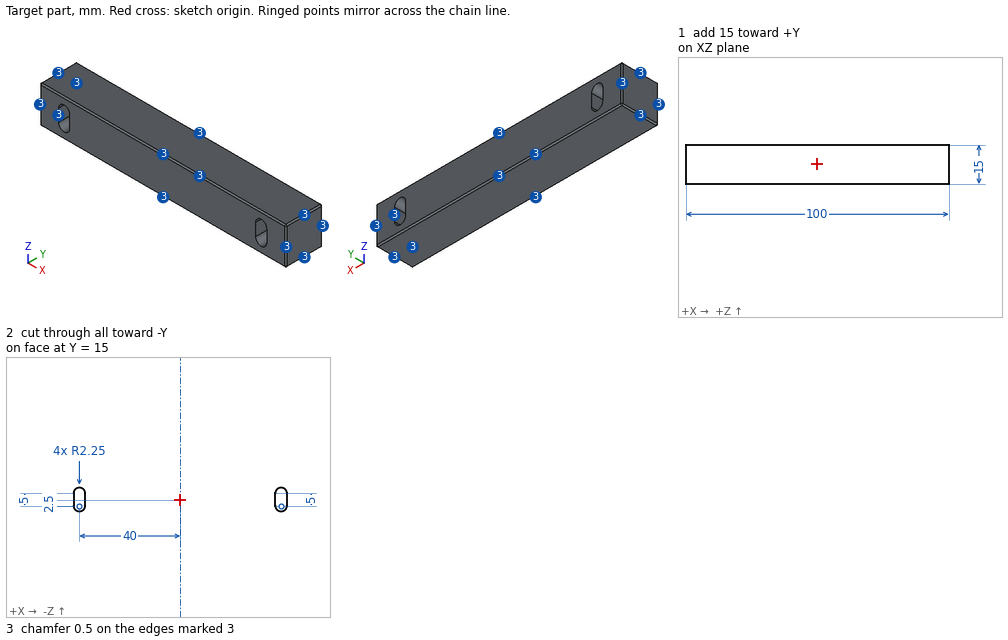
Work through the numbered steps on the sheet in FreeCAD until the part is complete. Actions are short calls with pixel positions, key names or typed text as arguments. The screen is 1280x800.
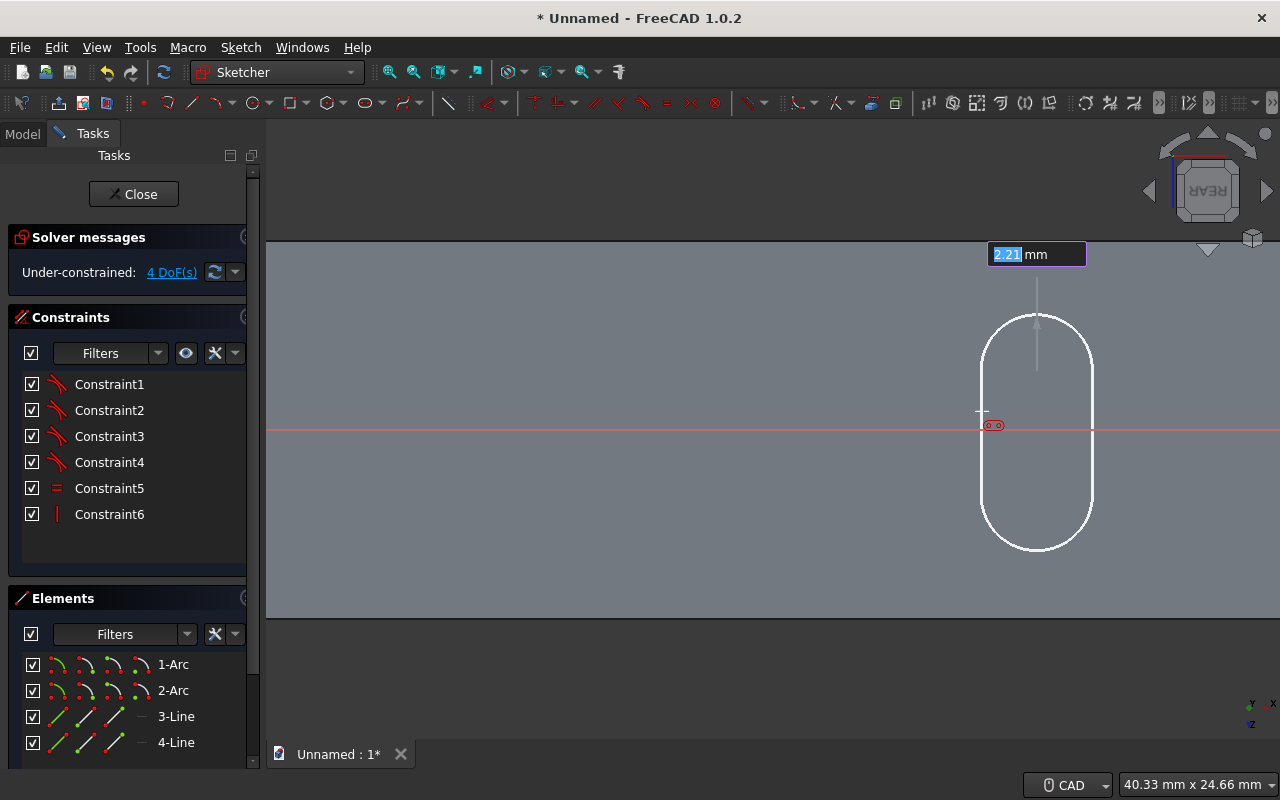
click(981, 411)
key(Escape)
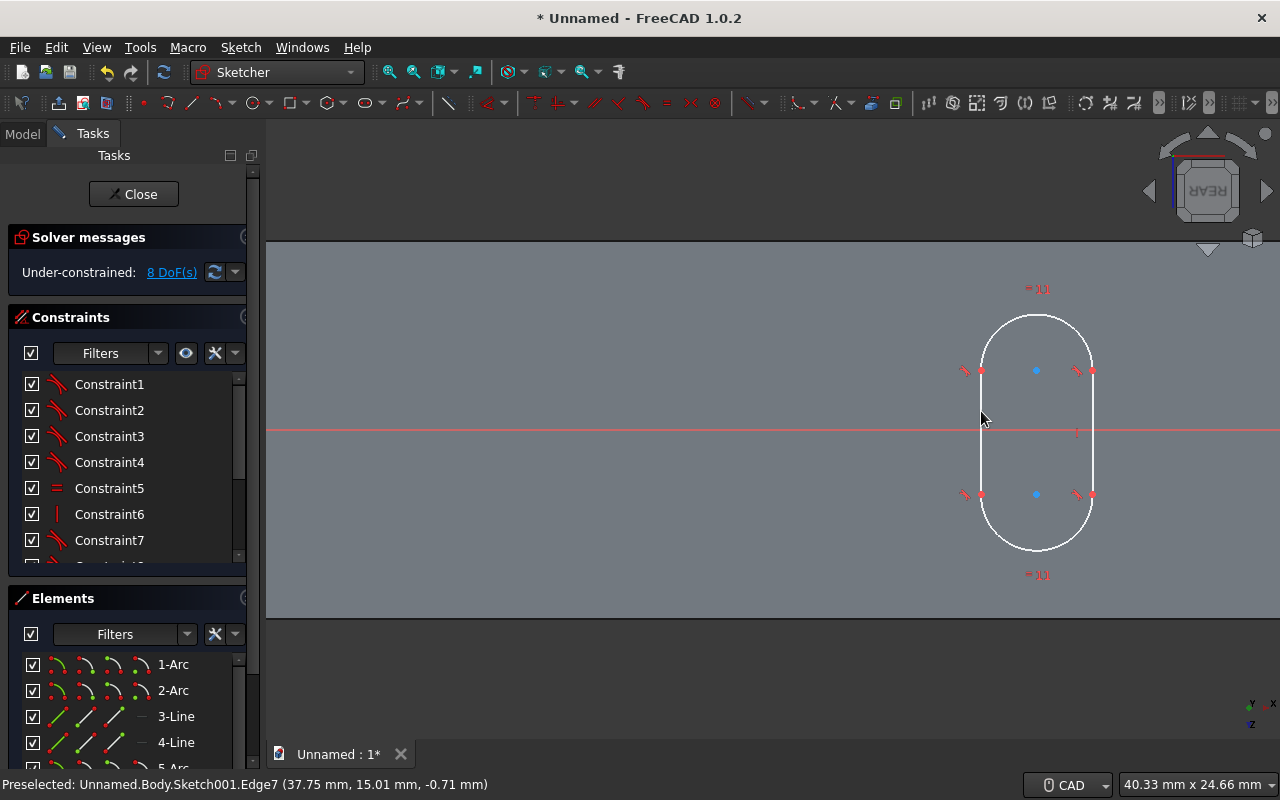
scroll(994, 429, down, 6)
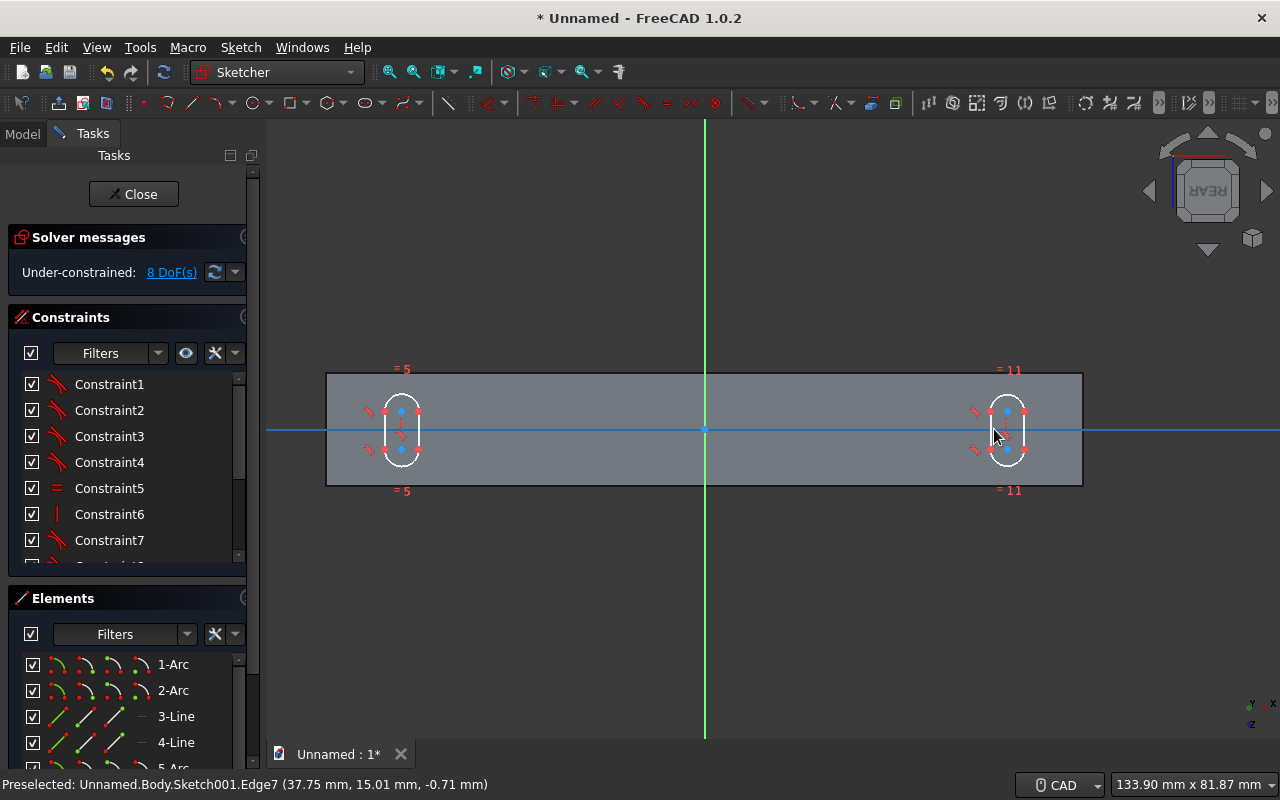
click(392, 463)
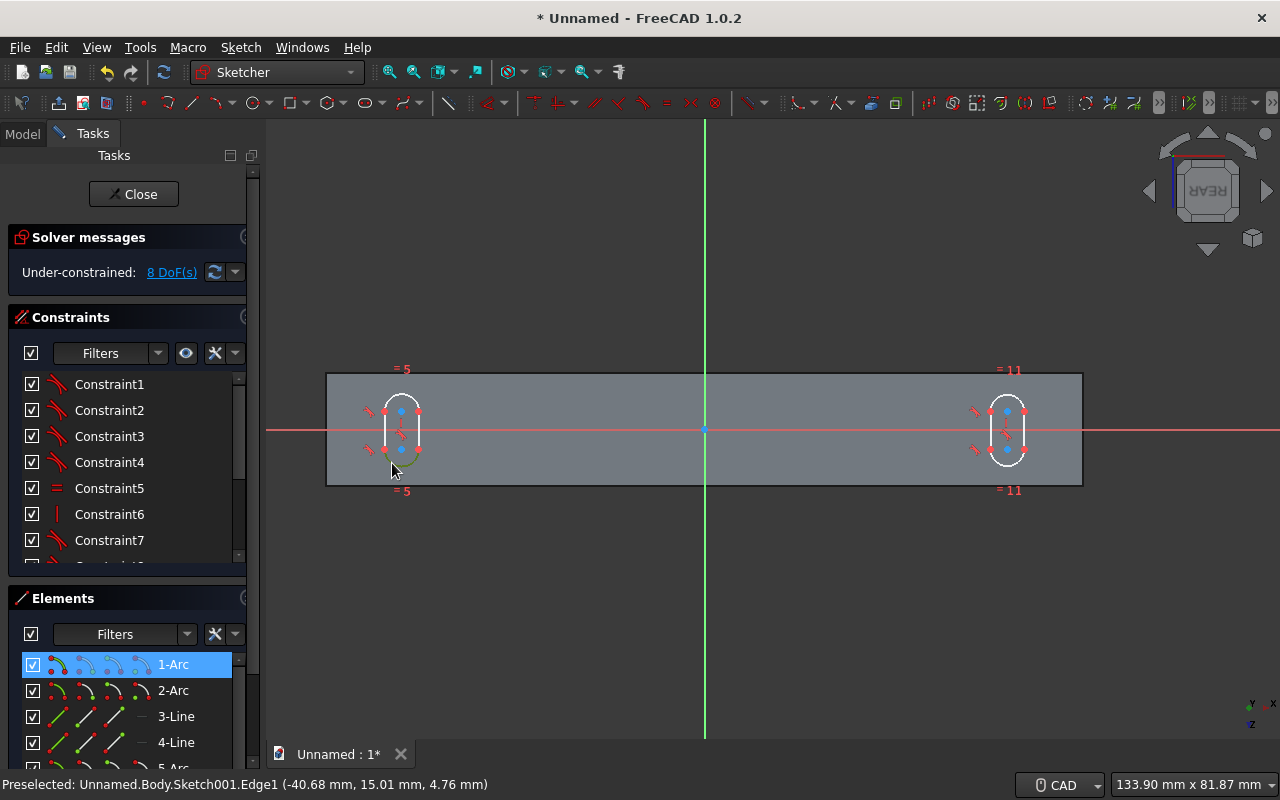
click(998, 463)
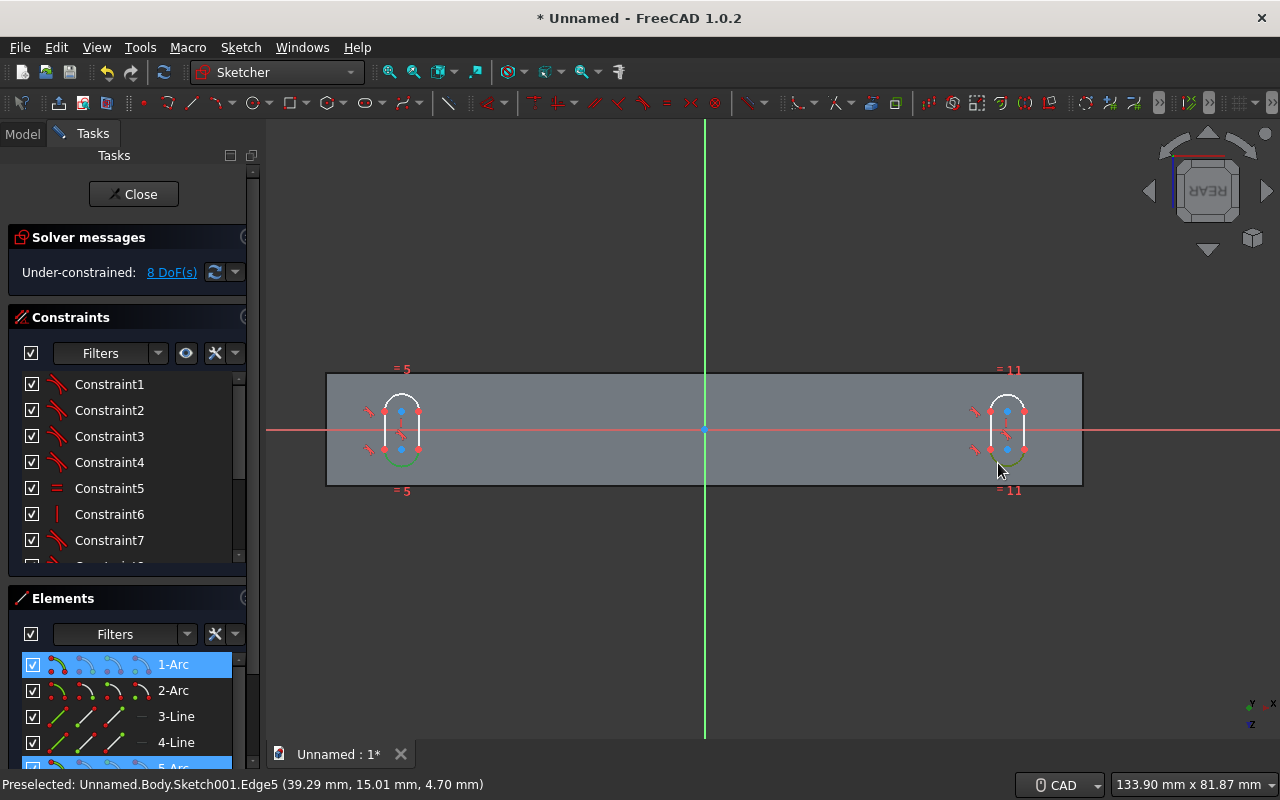
key(e)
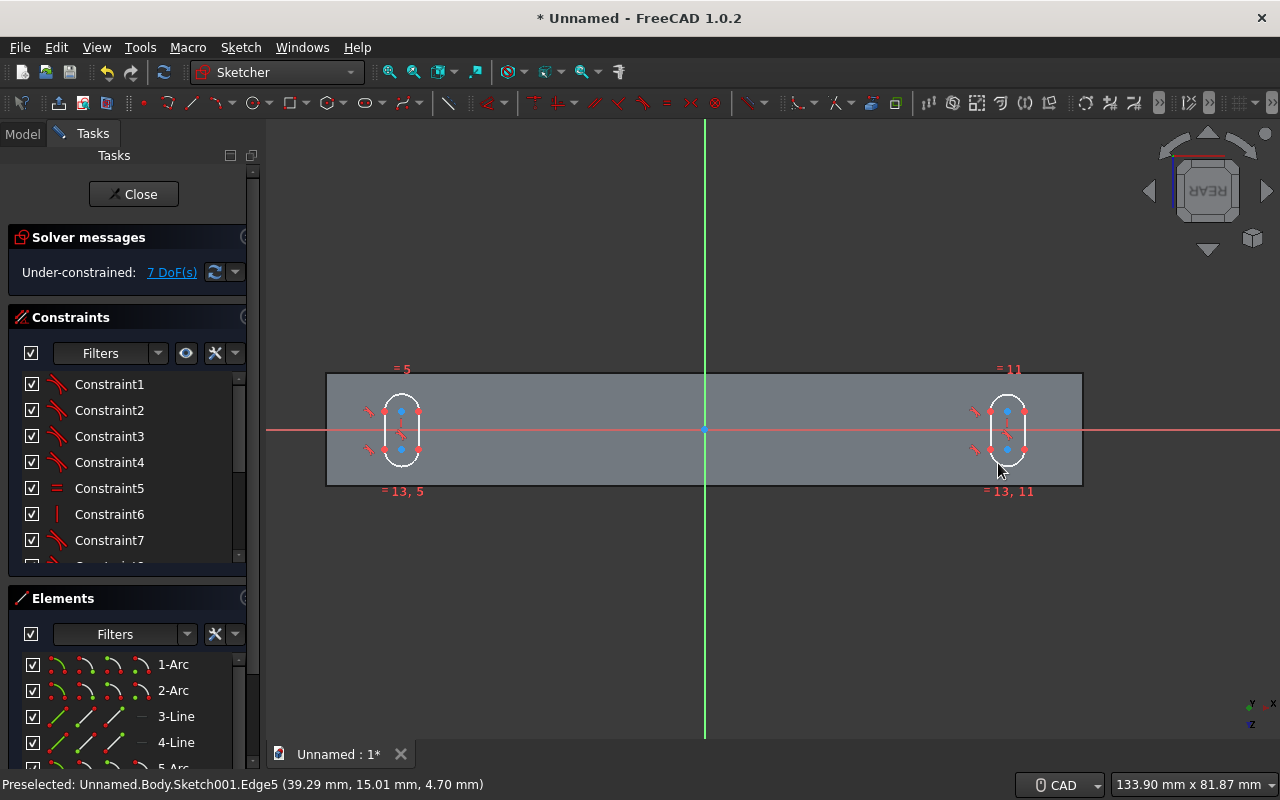
click(402, 449)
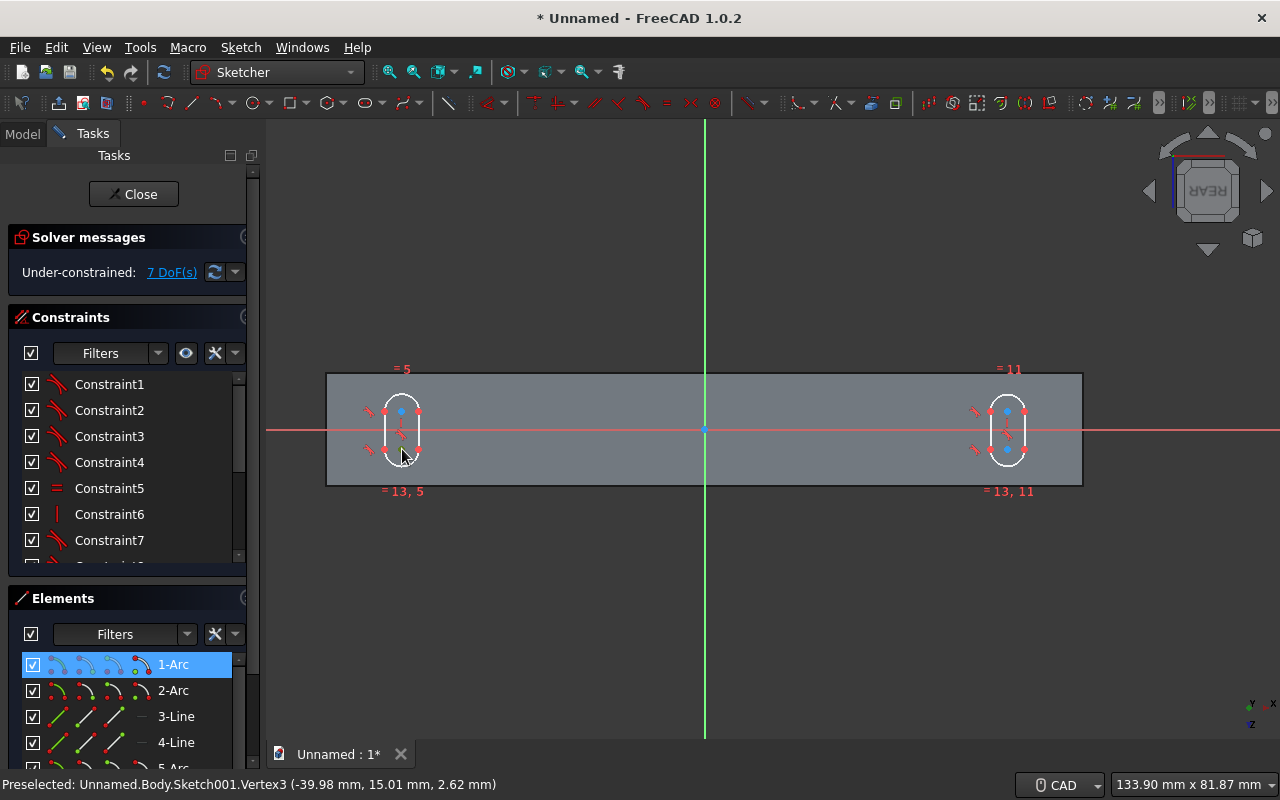
click(1008, 449)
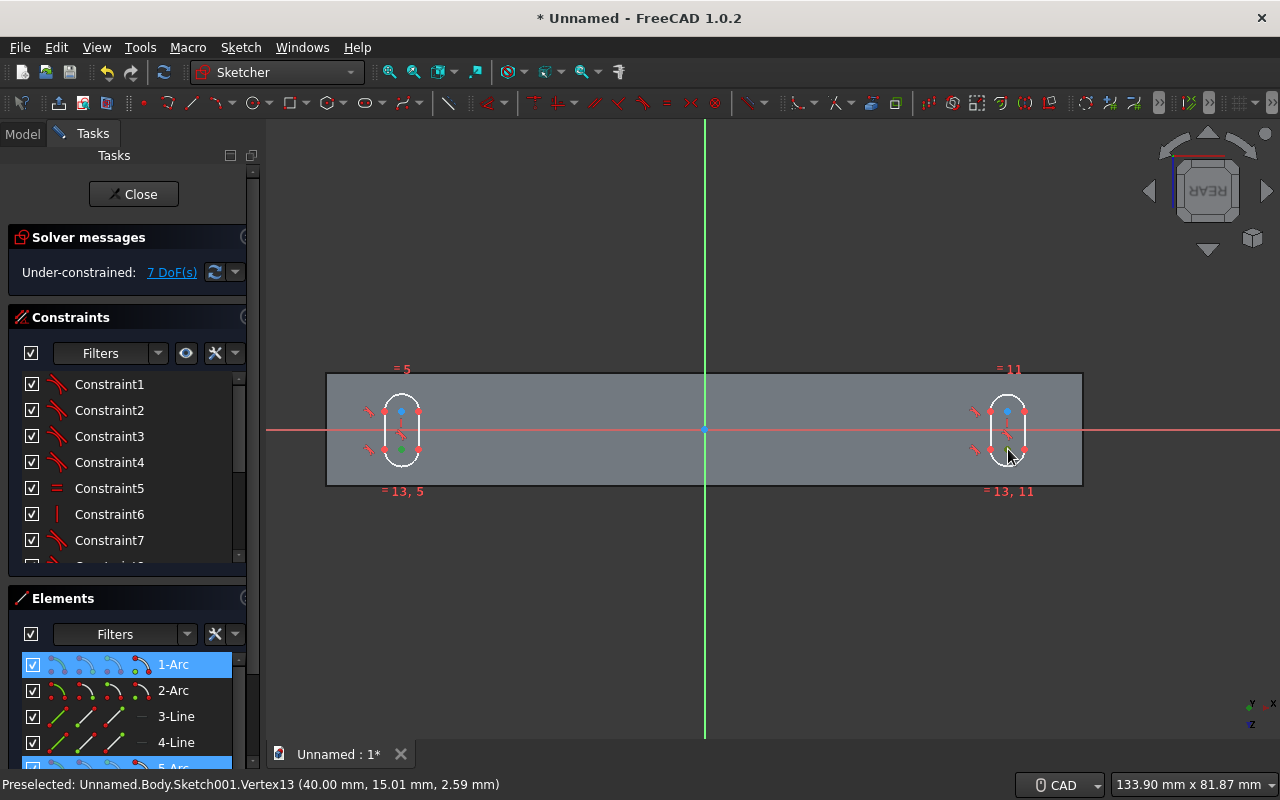
click(705, 671)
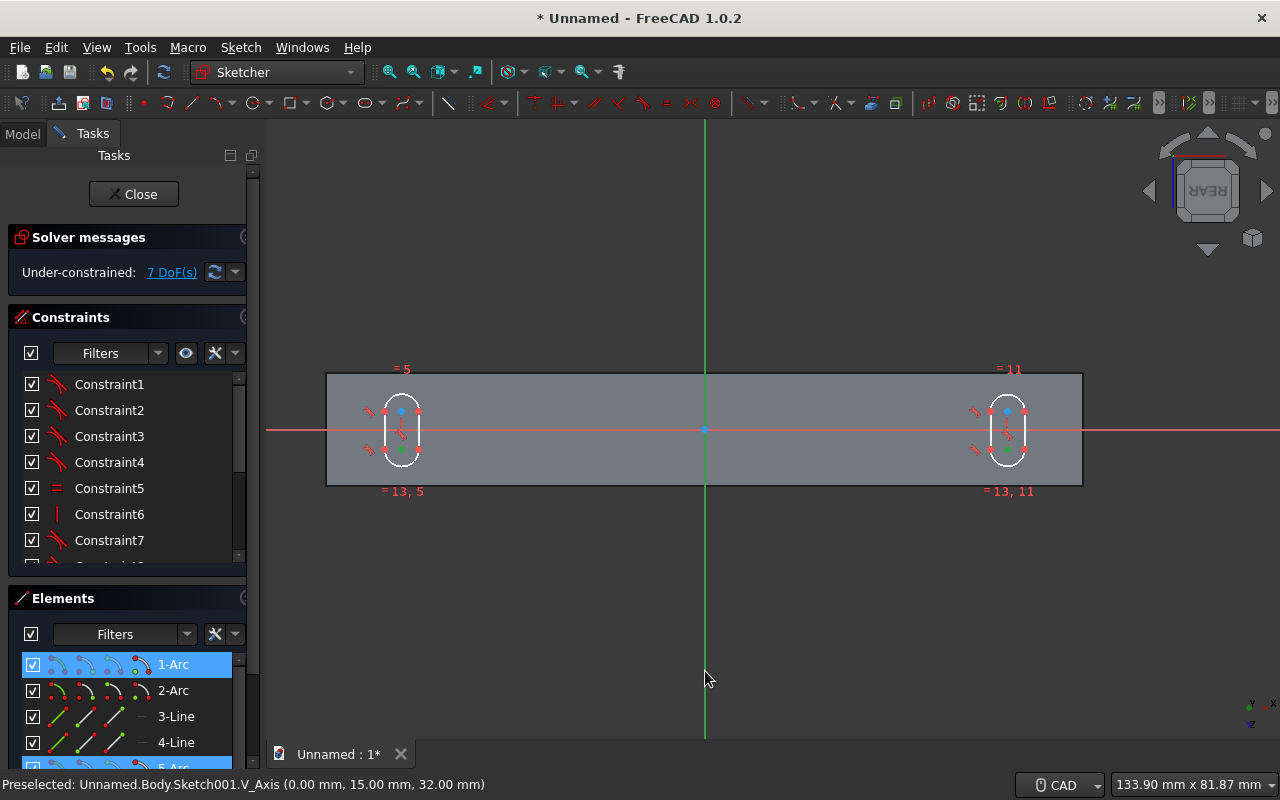
click(692, 104)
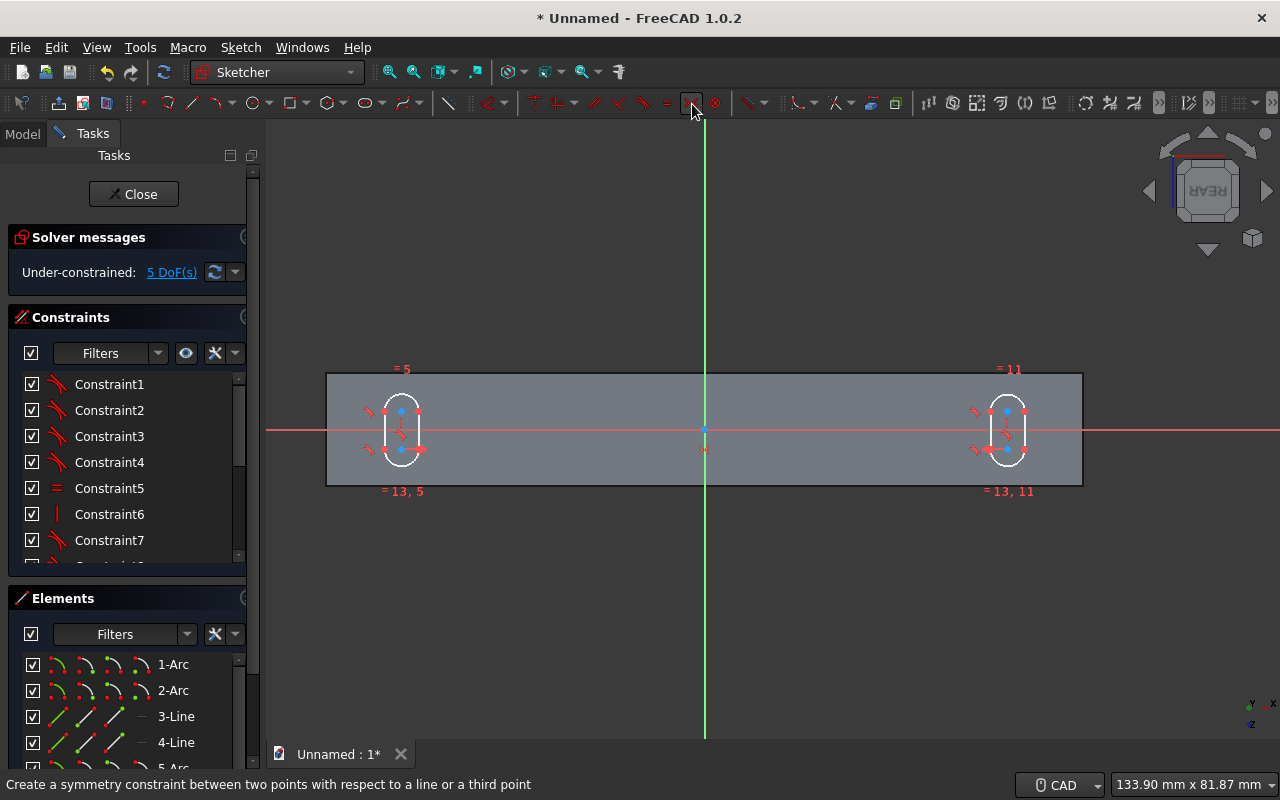
click(488, 104)